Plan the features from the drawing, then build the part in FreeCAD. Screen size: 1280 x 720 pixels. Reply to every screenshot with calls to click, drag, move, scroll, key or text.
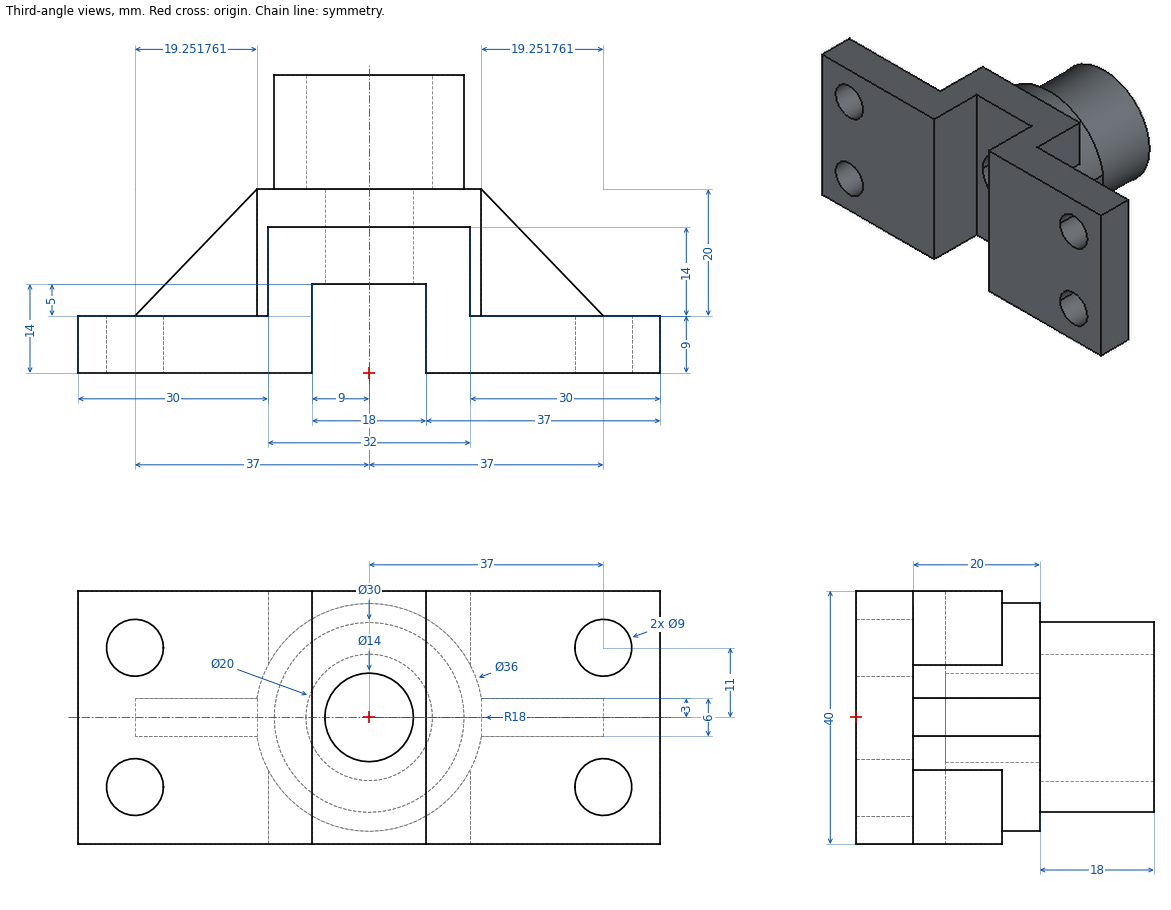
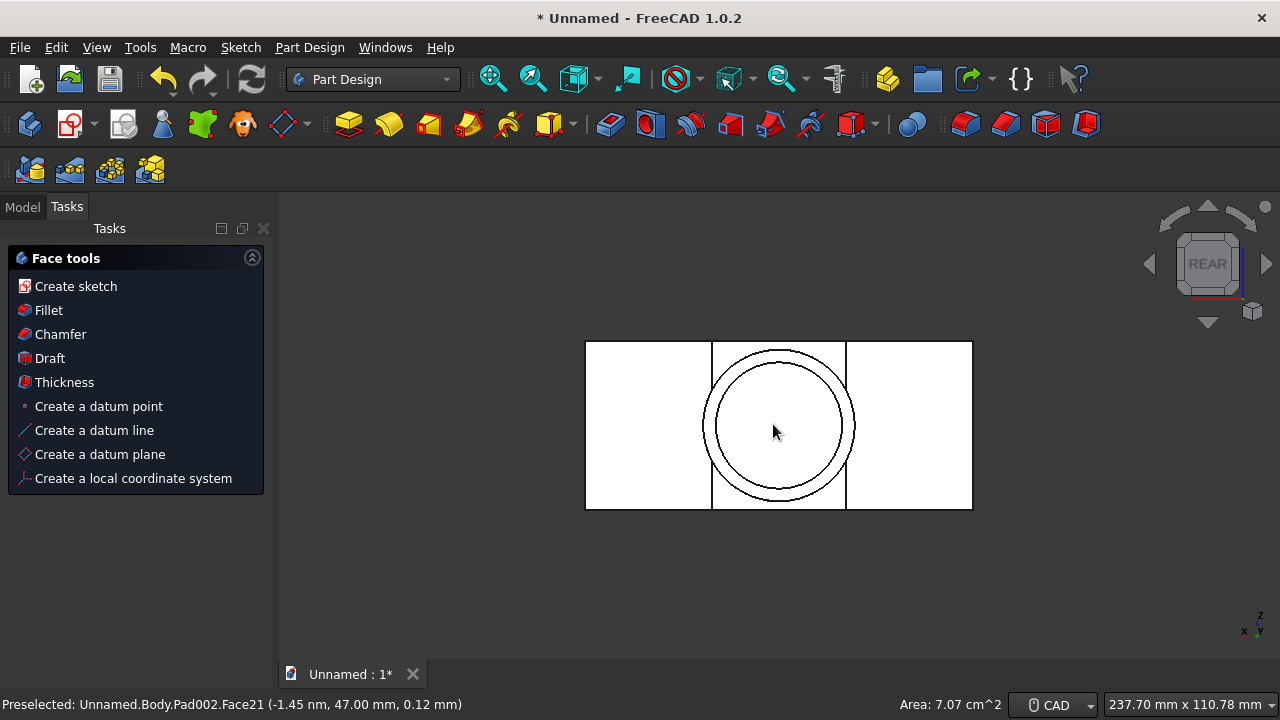
click(70, 124)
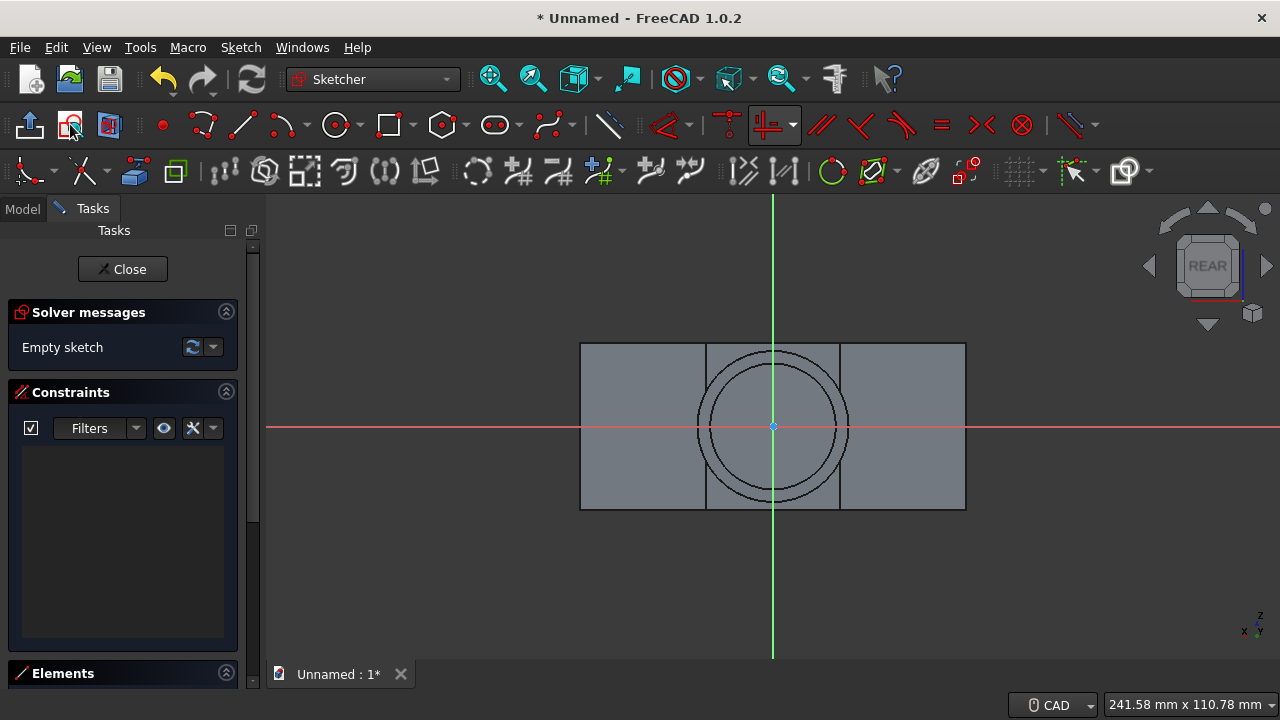
scroll(803, 427, up, 6)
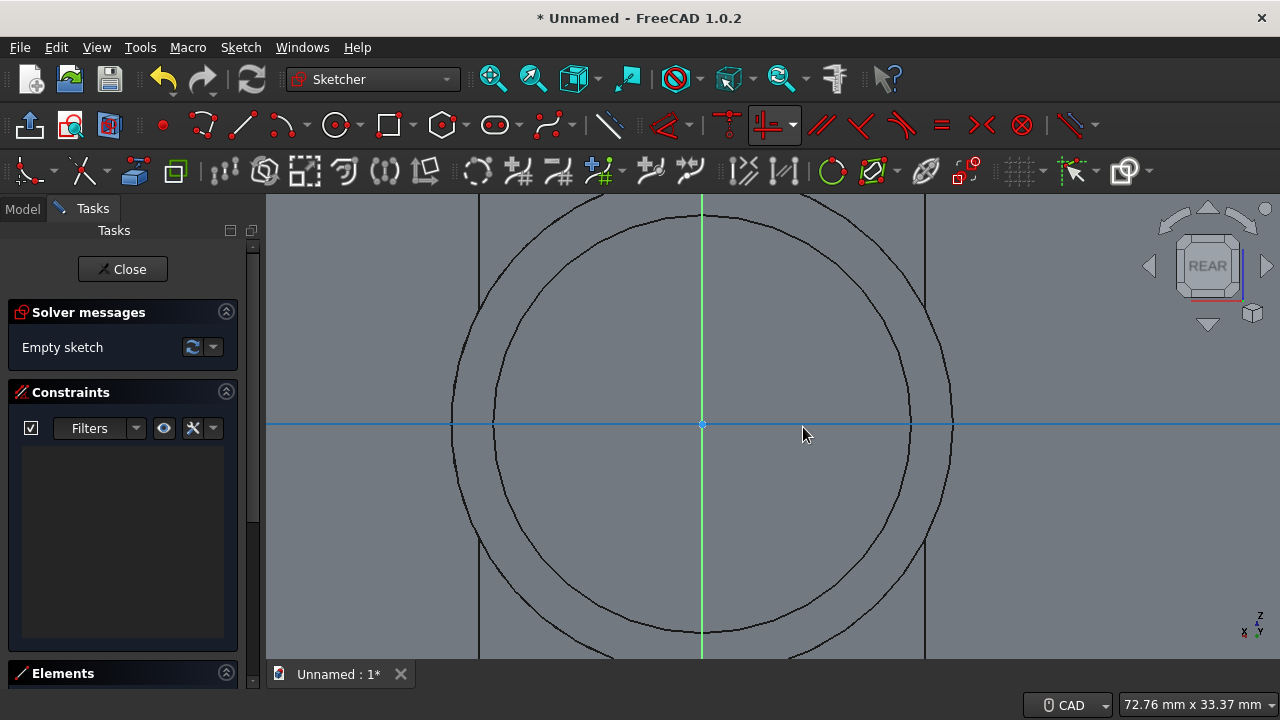
key(g)
key(c)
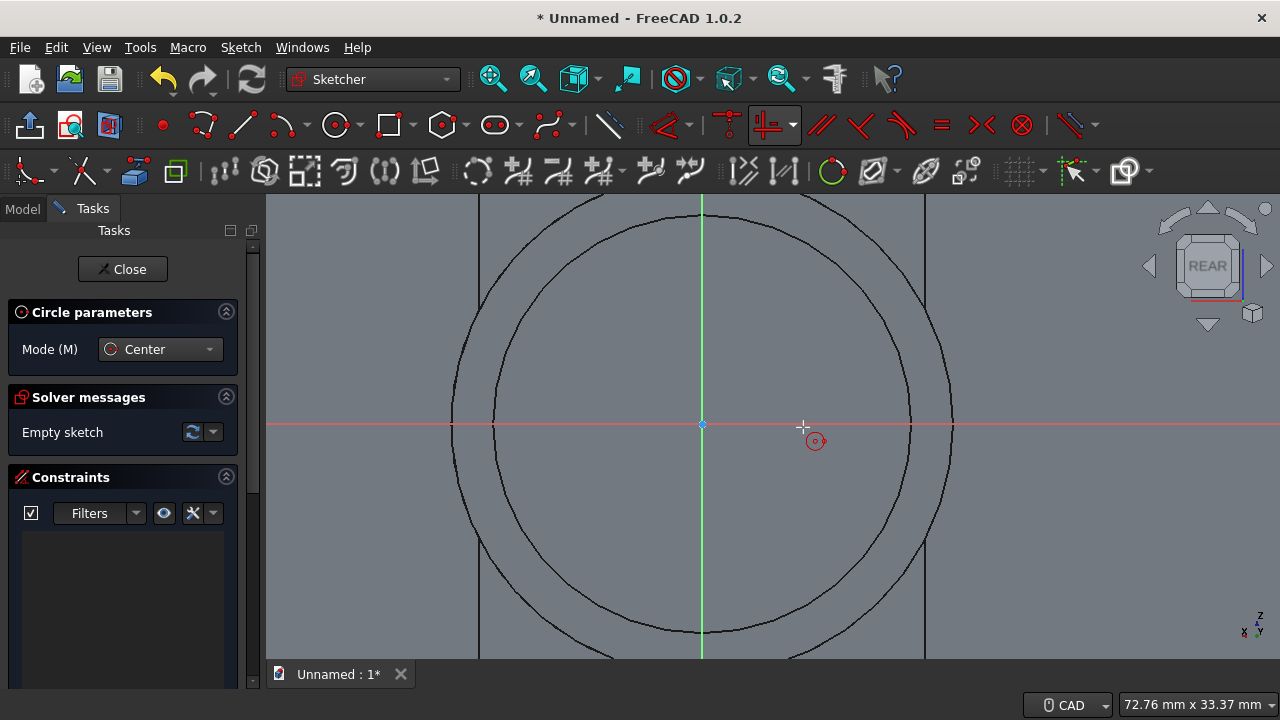
click(702, 424)
click(801, 326)
key(Escape)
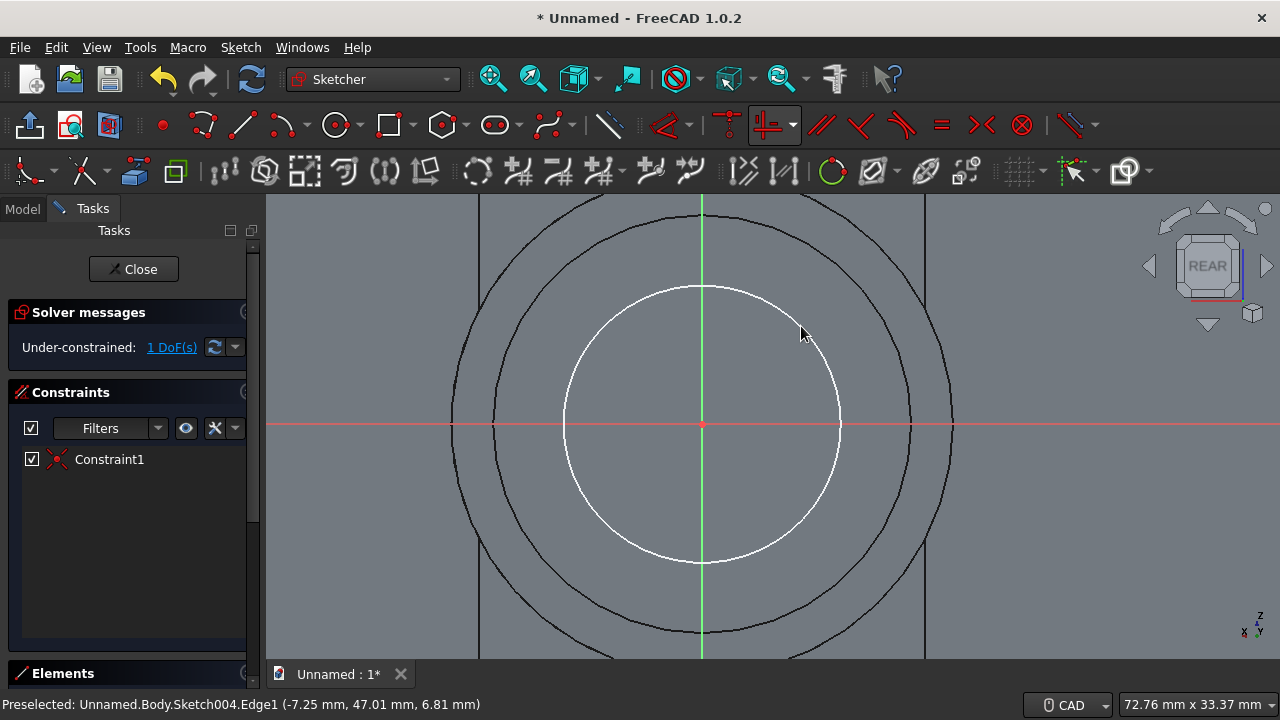
key(d)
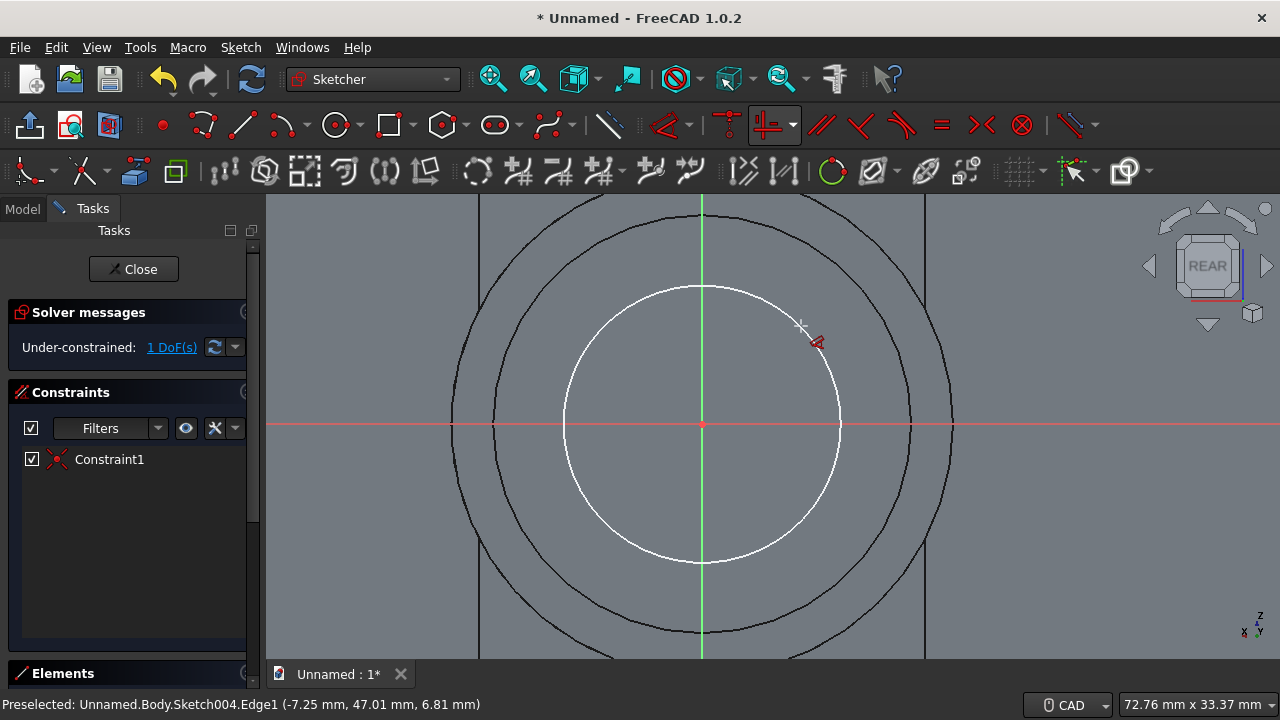
click(800, 326)
click(823, 303)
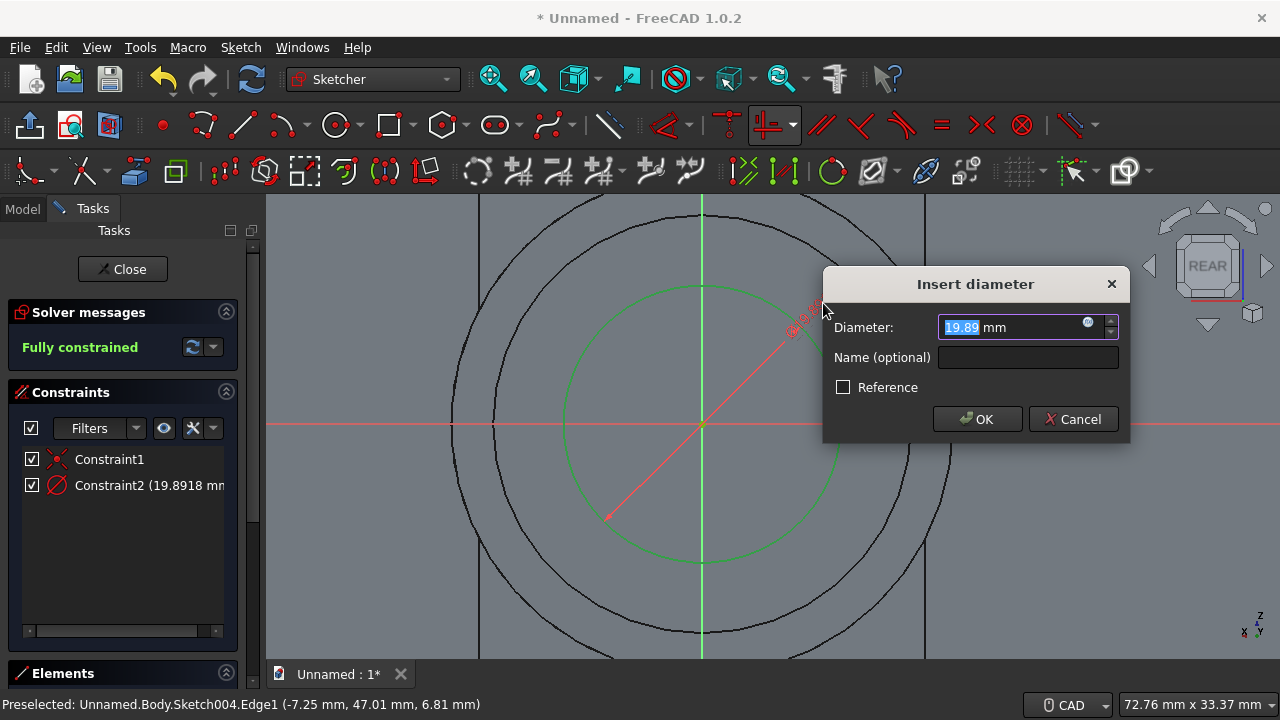
text(20)
key(Return)
key(Escape)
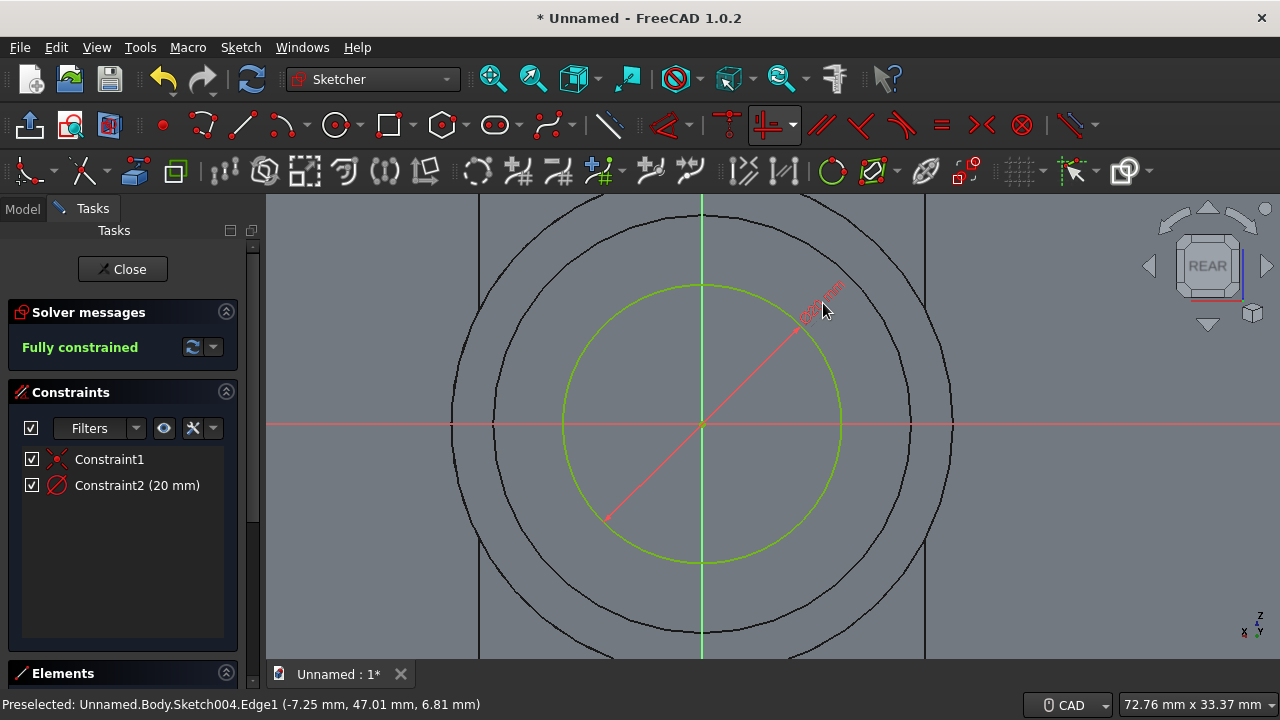
click(123, 269)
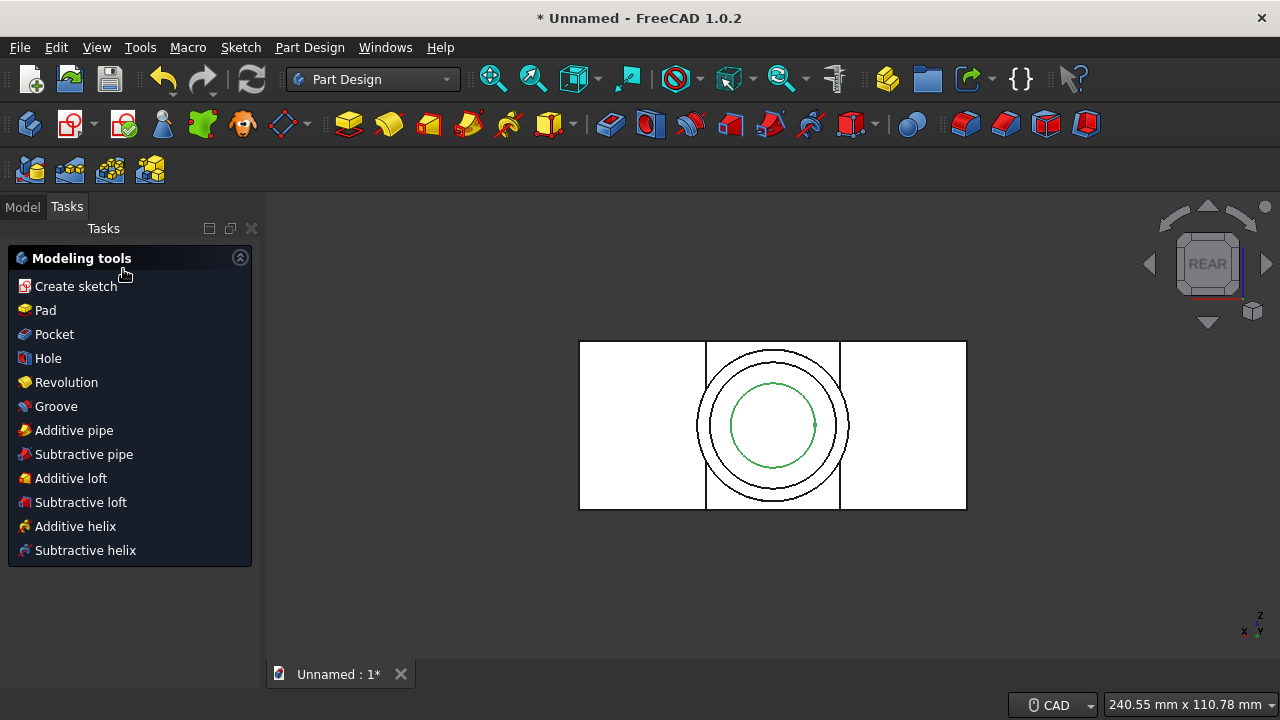
click(612, 124)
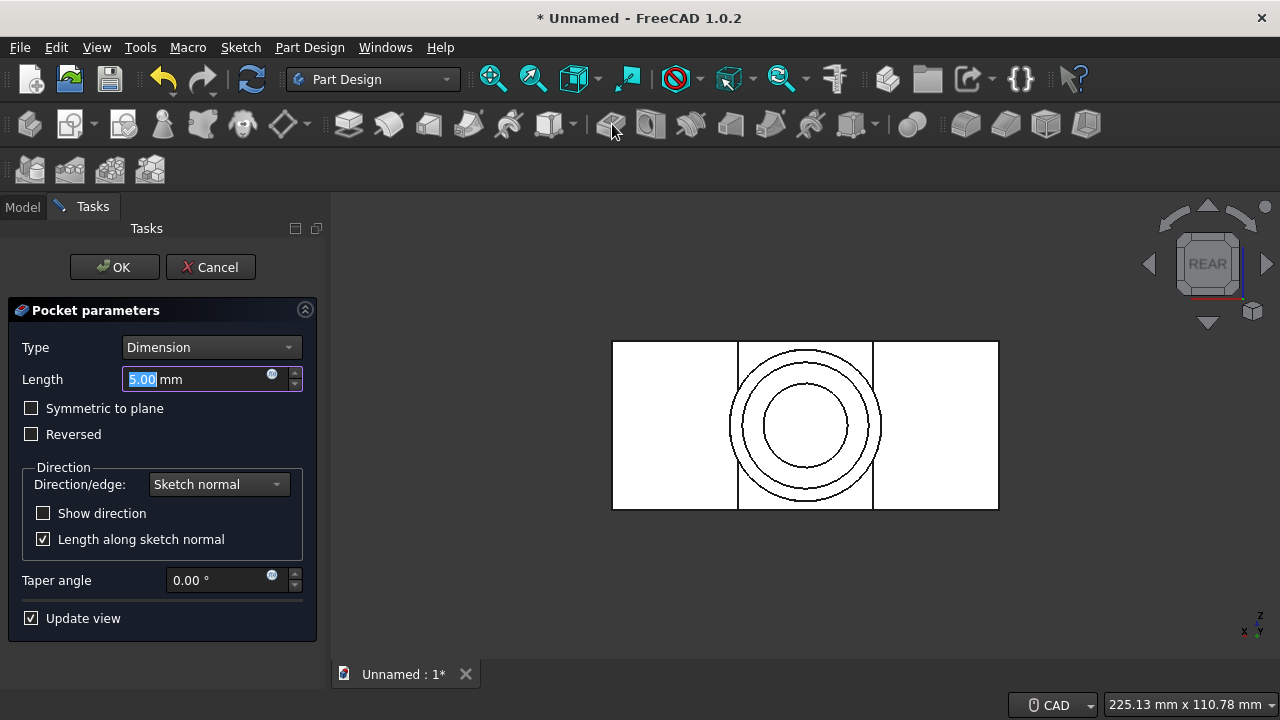
text(18)
key(Tab)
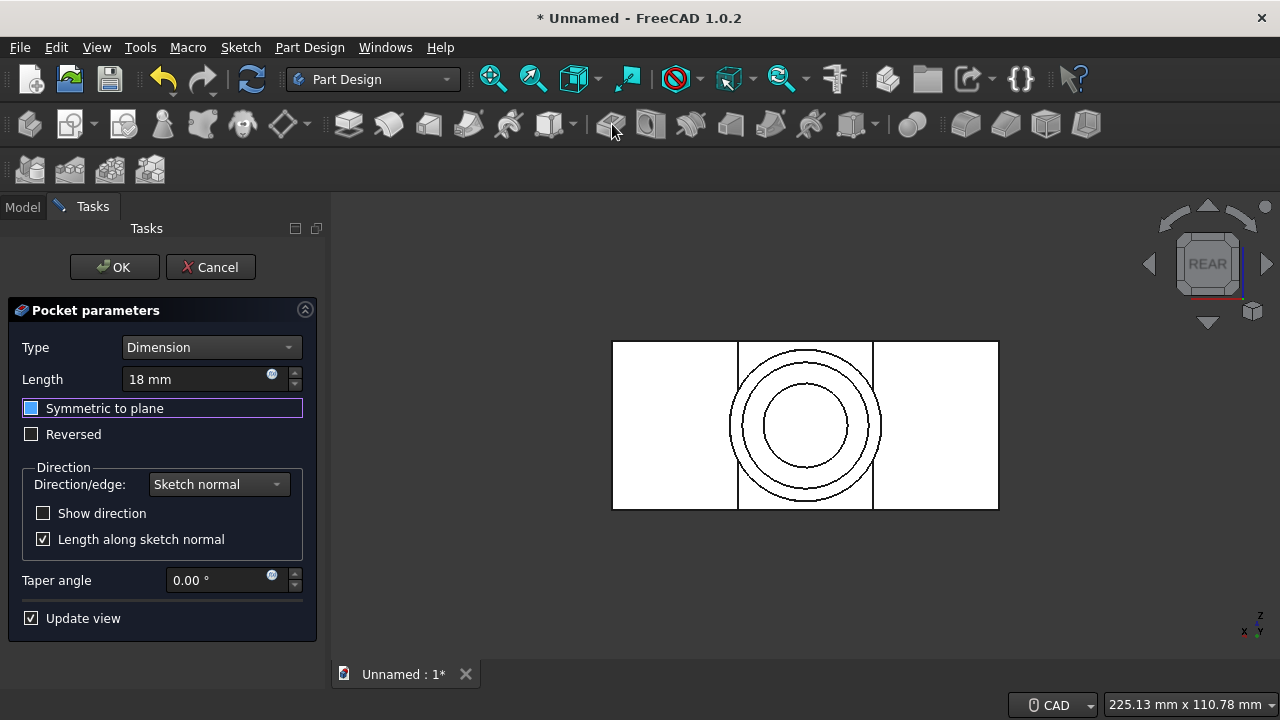
click(115, 267)